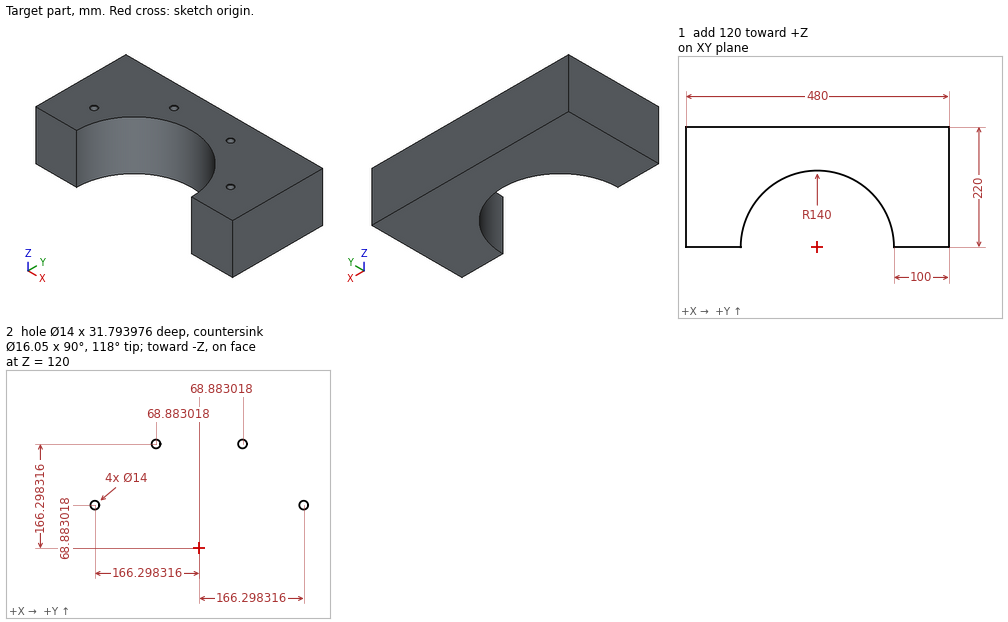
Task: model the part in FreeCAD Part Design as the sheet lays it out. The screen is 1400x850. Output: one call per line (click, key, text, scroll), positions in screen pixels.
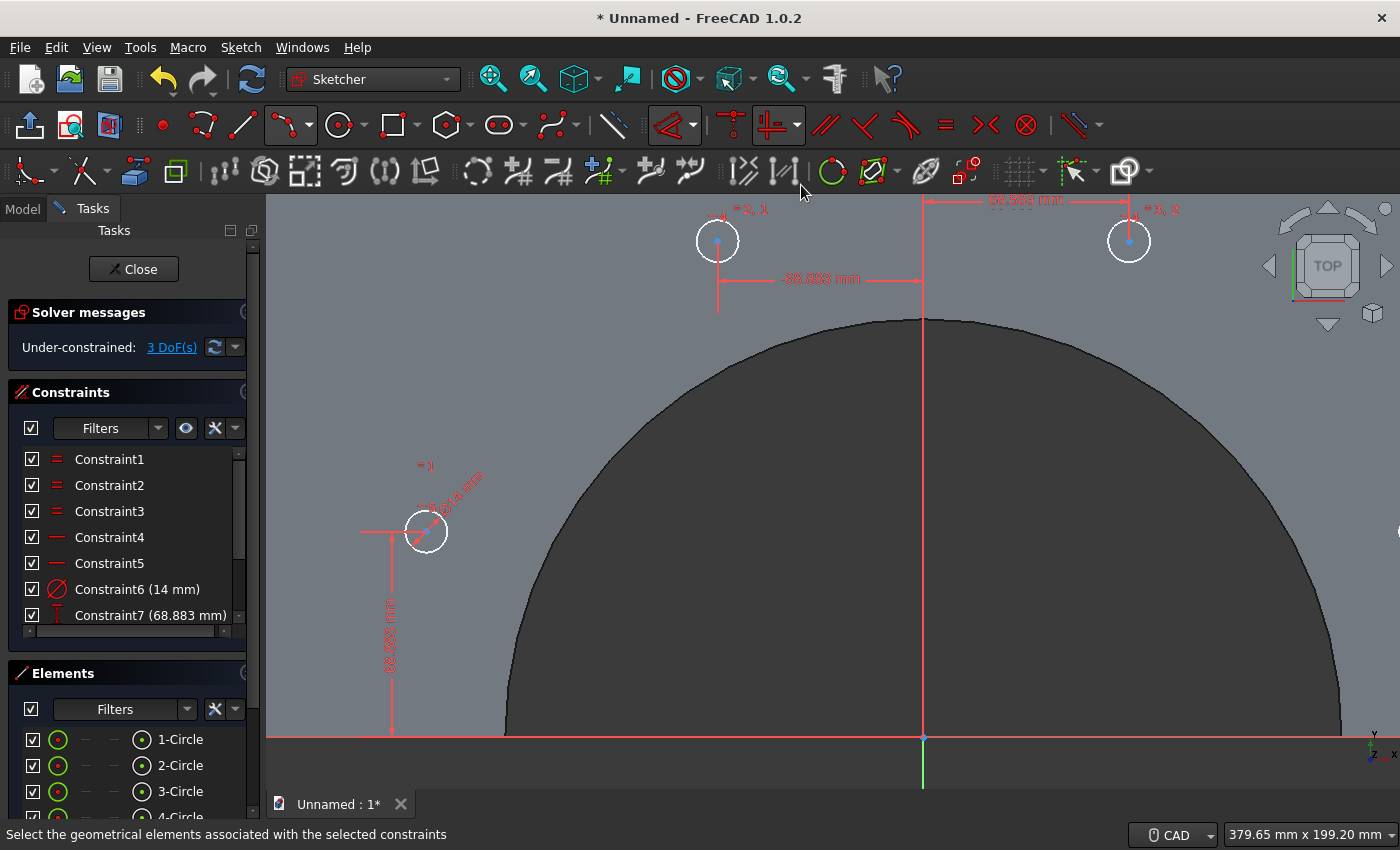
click(426, 532)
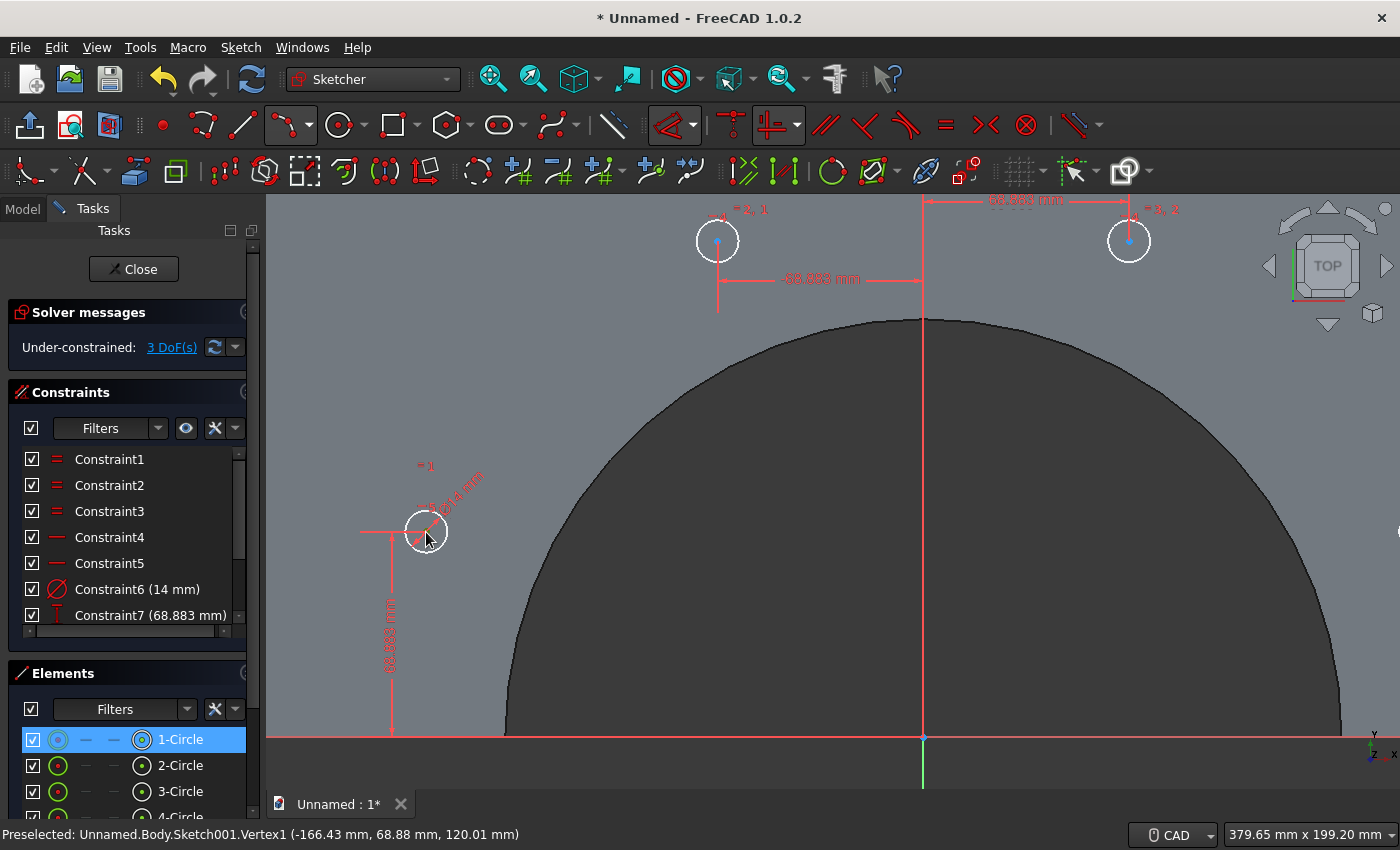
key(l)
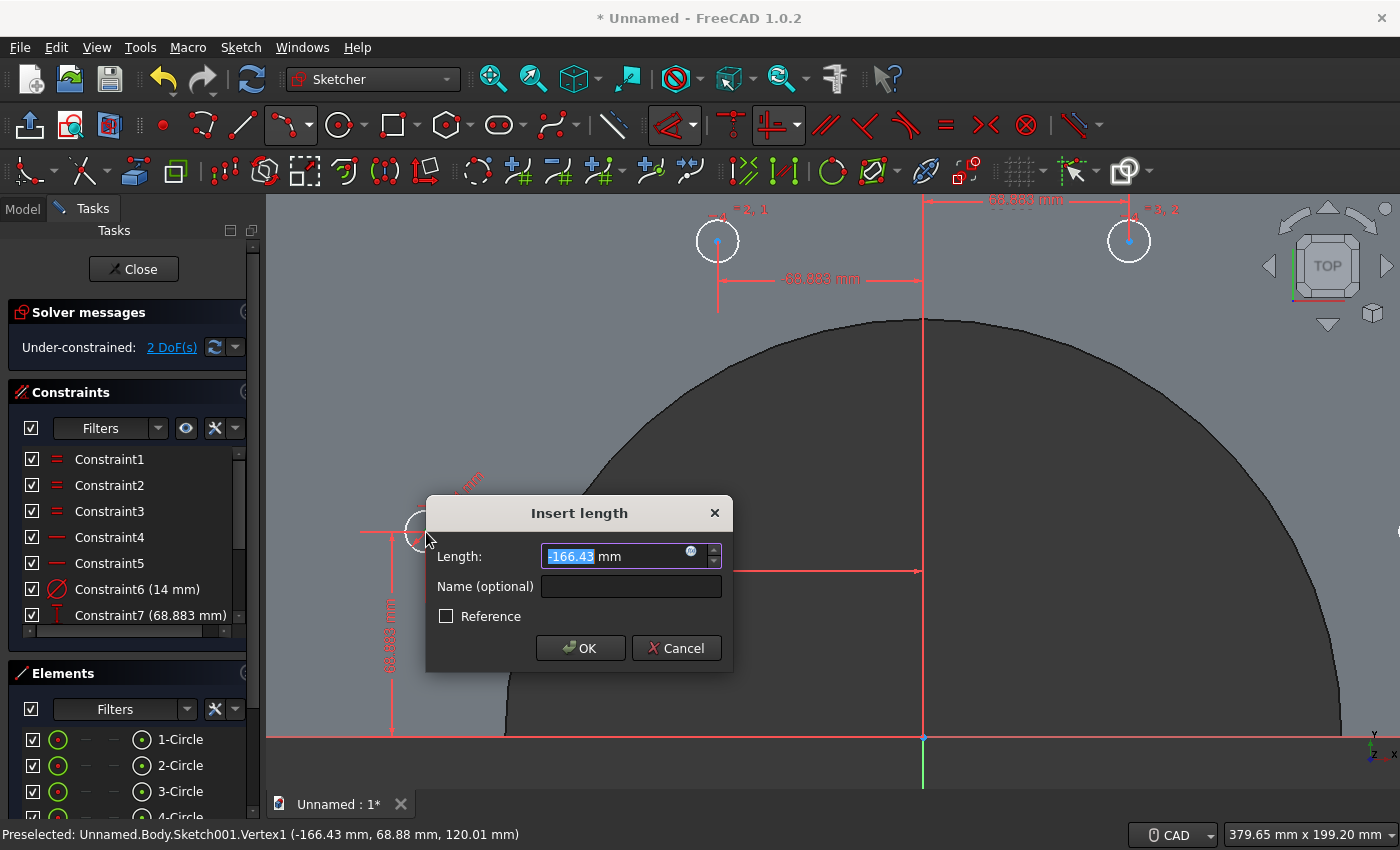
text(-166.298316)
key(Return)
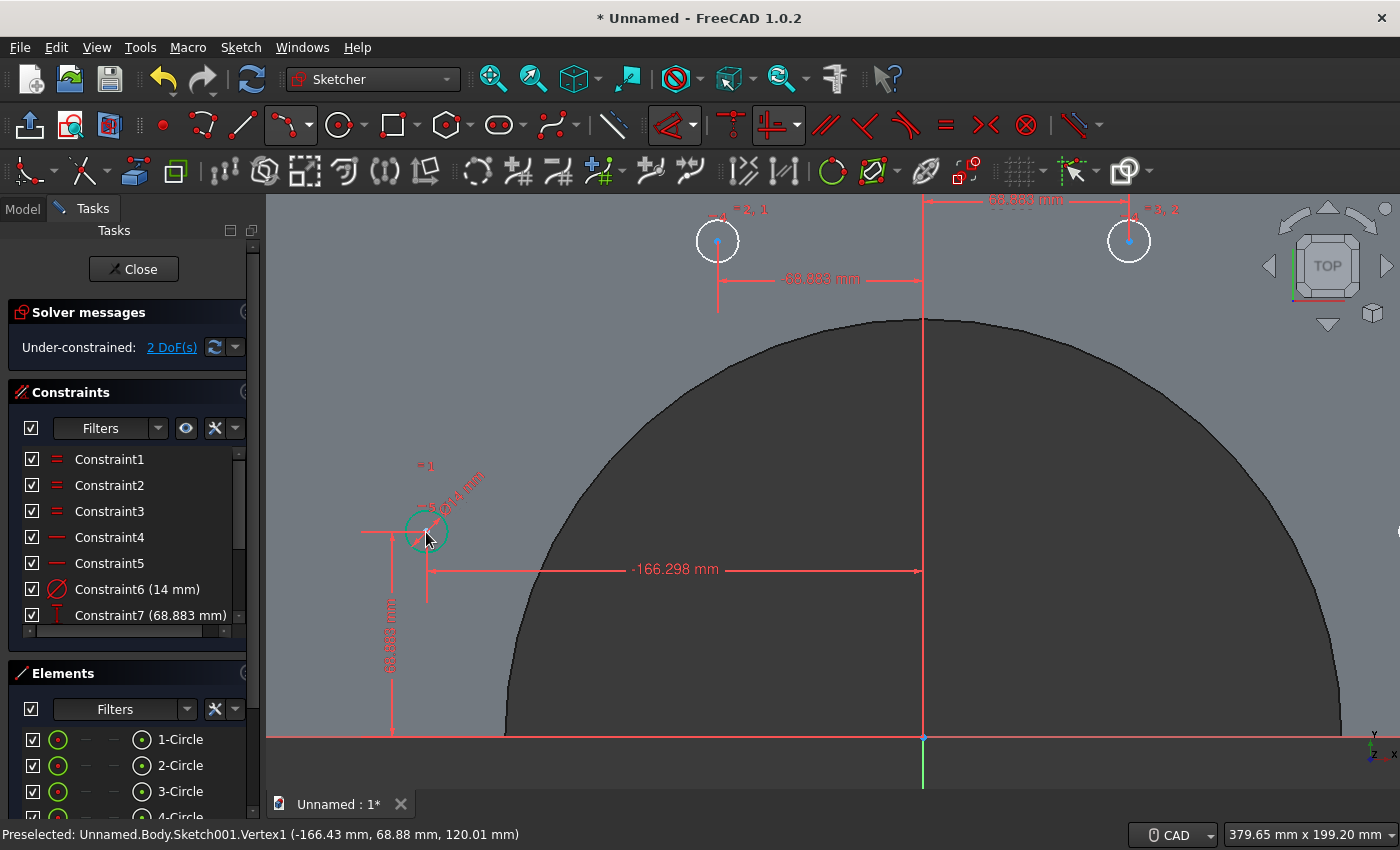
click(718, 241)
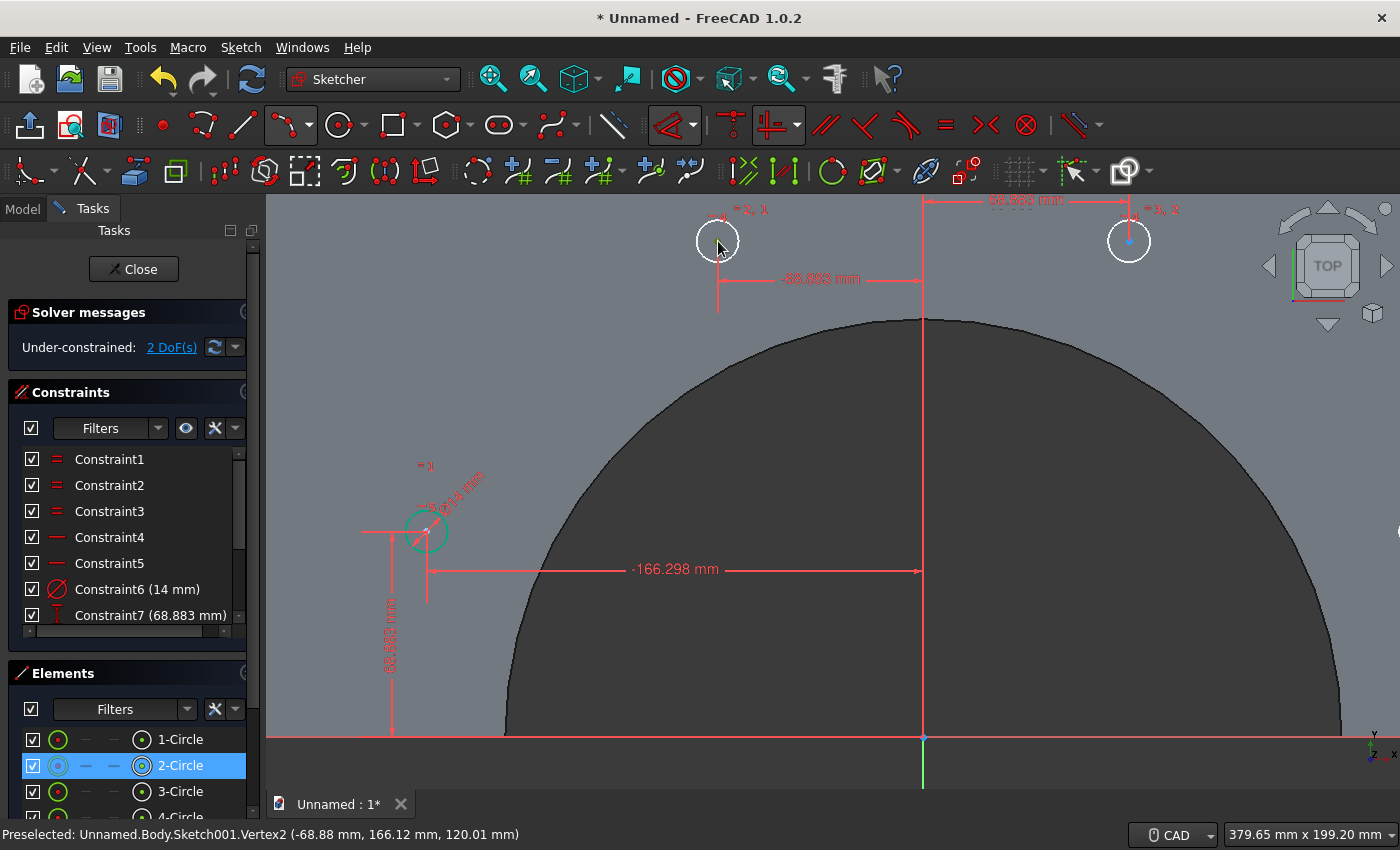
key(i)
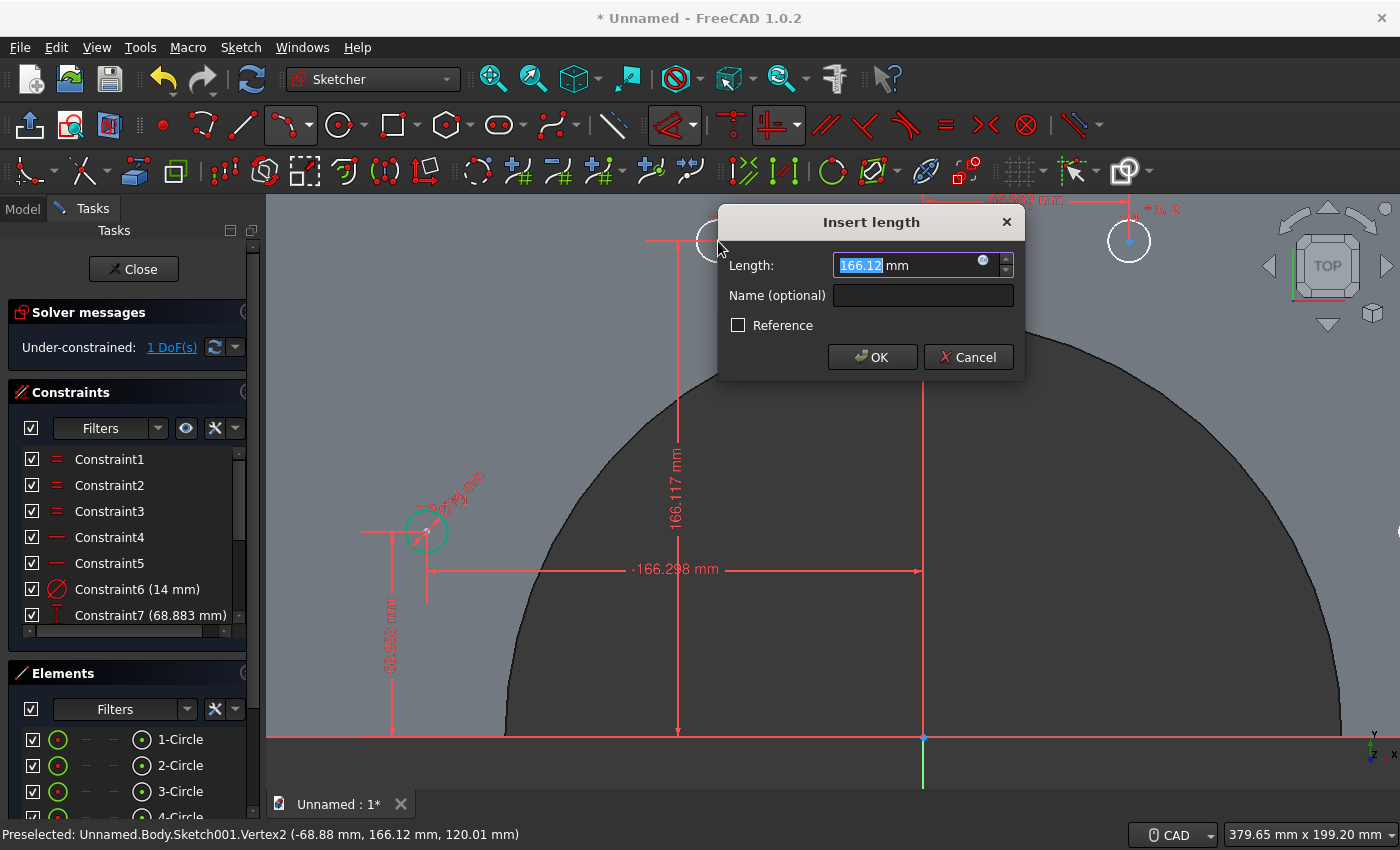
text(166.298316)
key(Return)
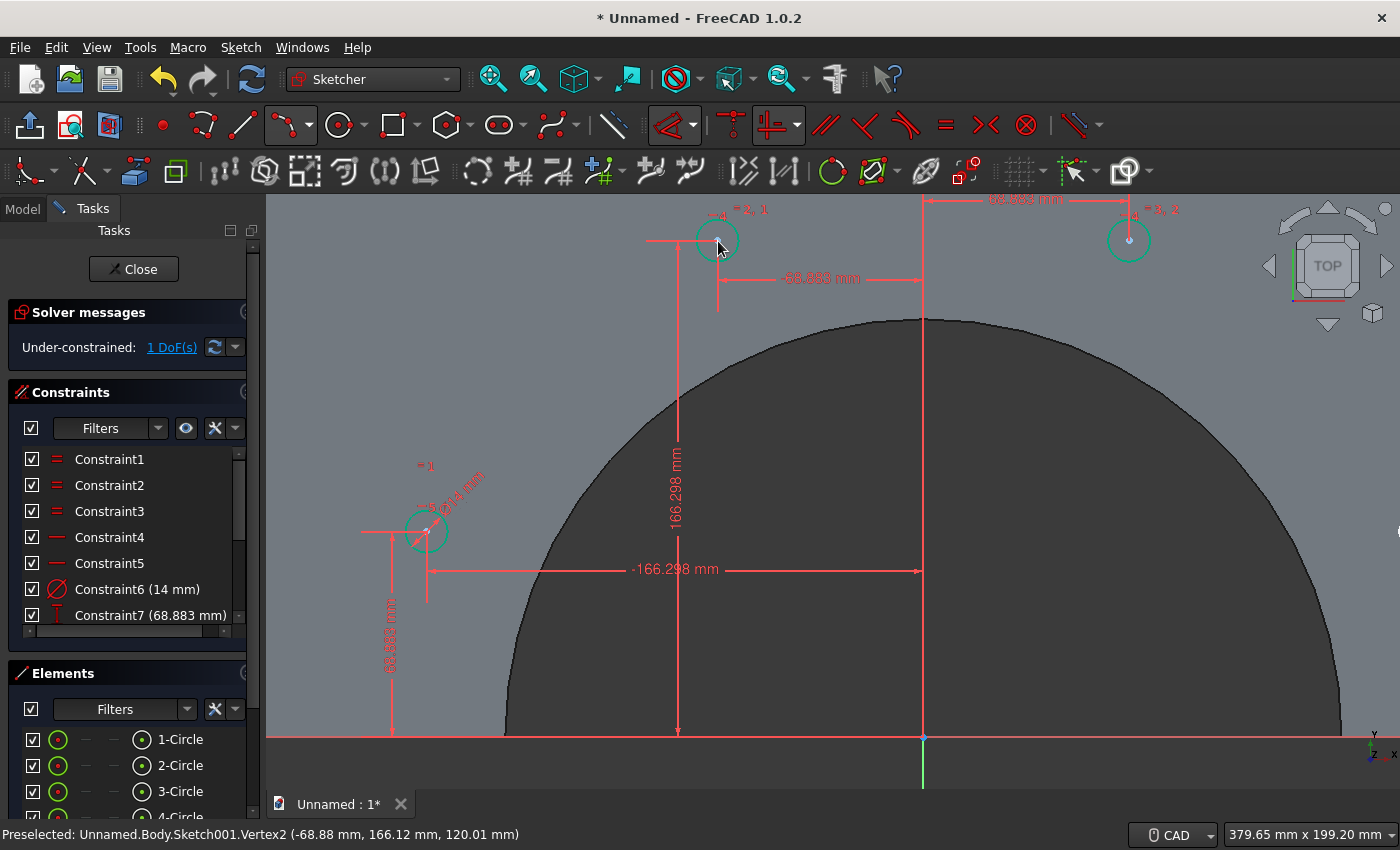
scroll(441, 518, down, 2)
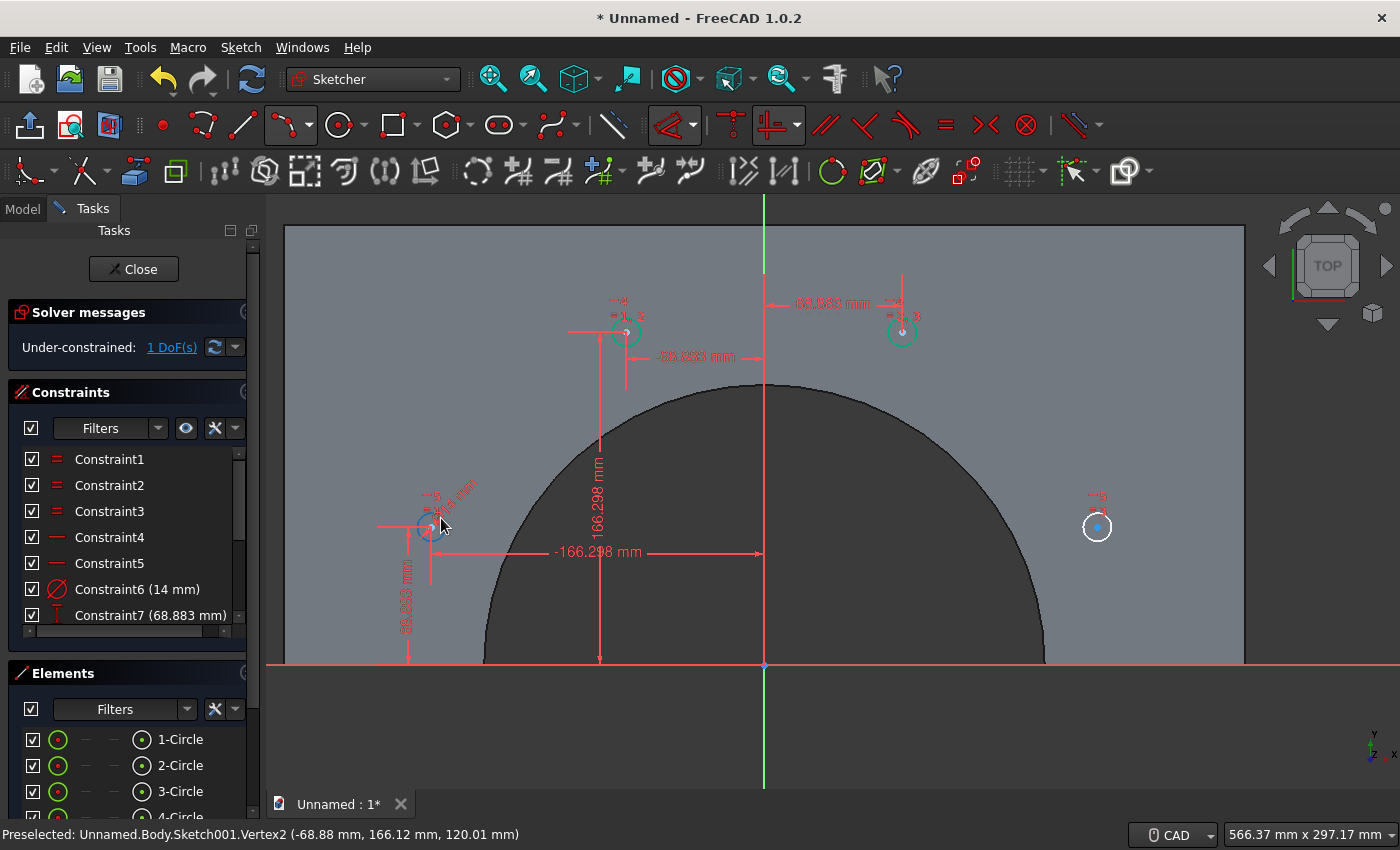
click(1097, 527)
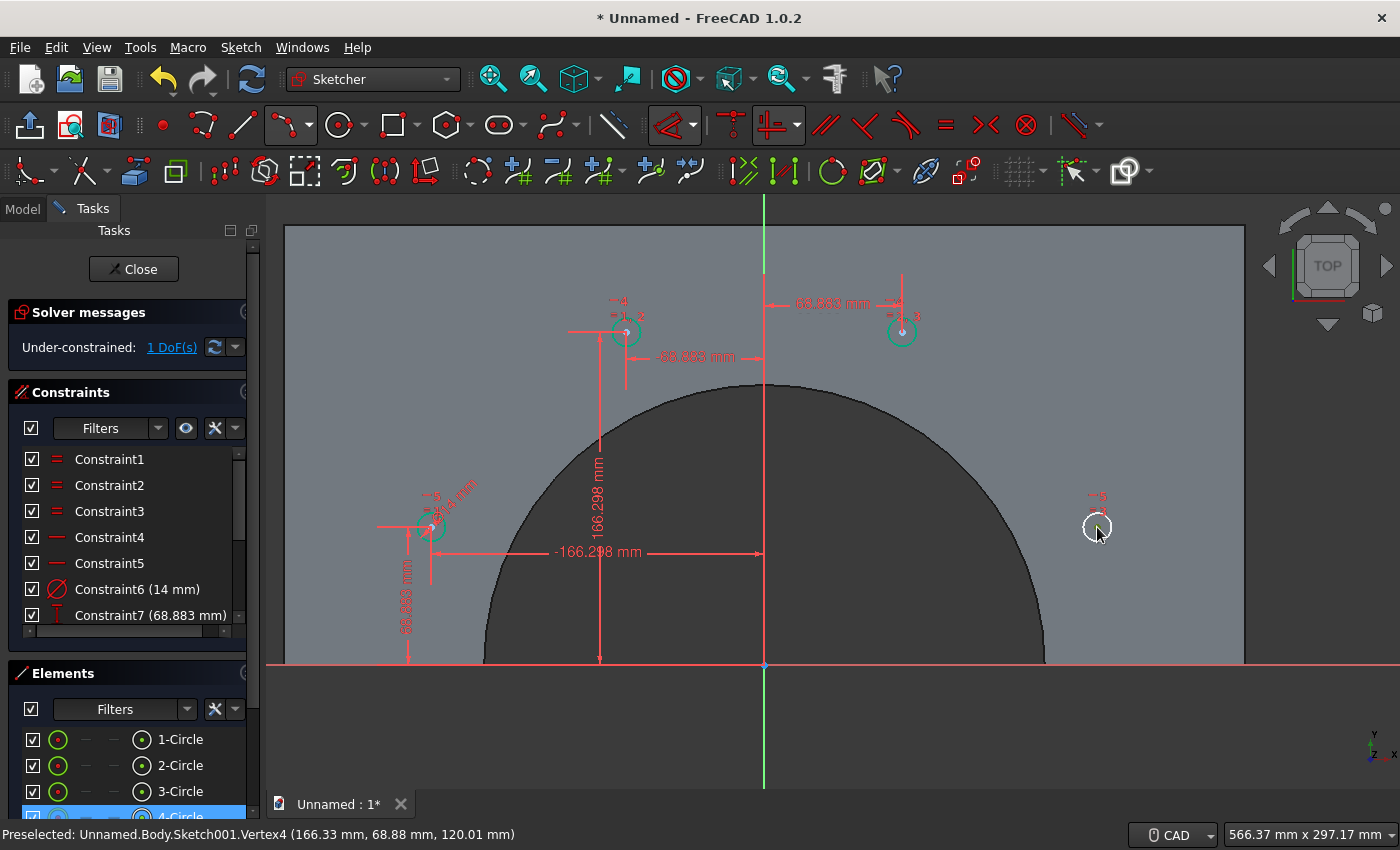
click(696, 126)